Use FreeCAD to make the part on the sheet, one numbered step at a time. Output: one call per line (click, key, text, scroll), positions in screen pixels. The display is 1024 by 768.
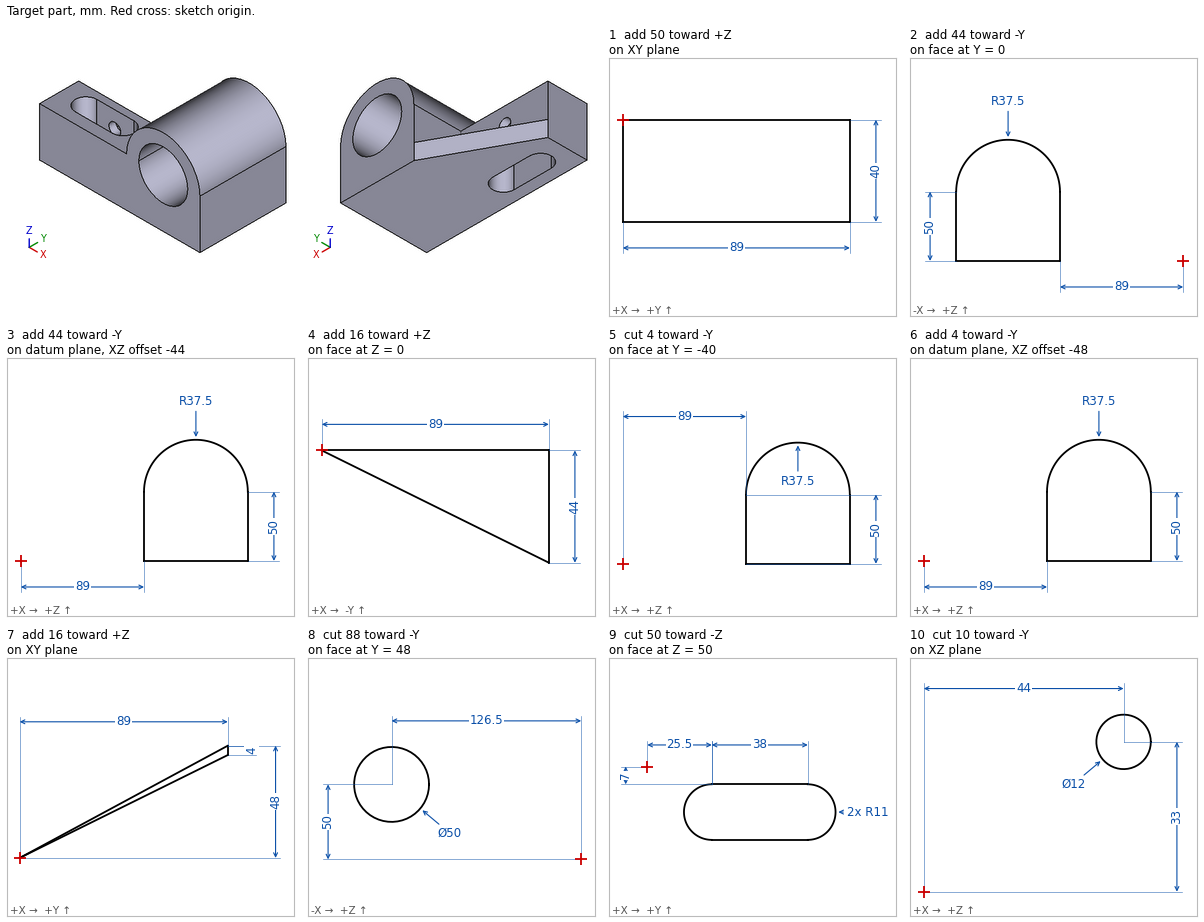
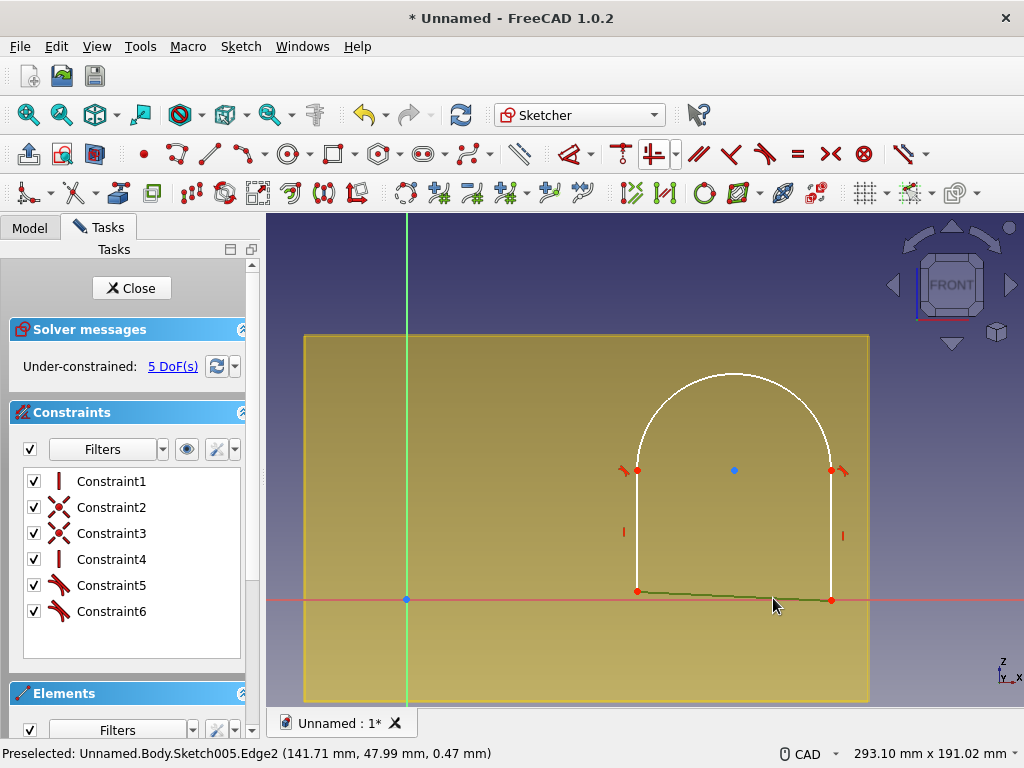
click(676, 154)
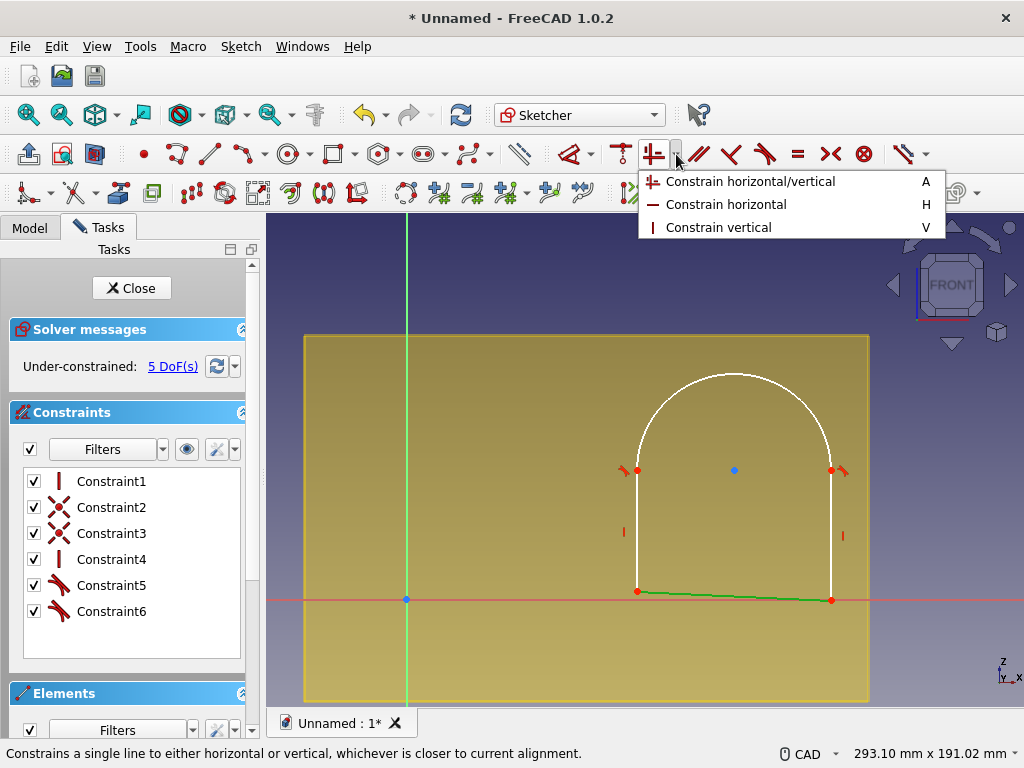
click(792, 204)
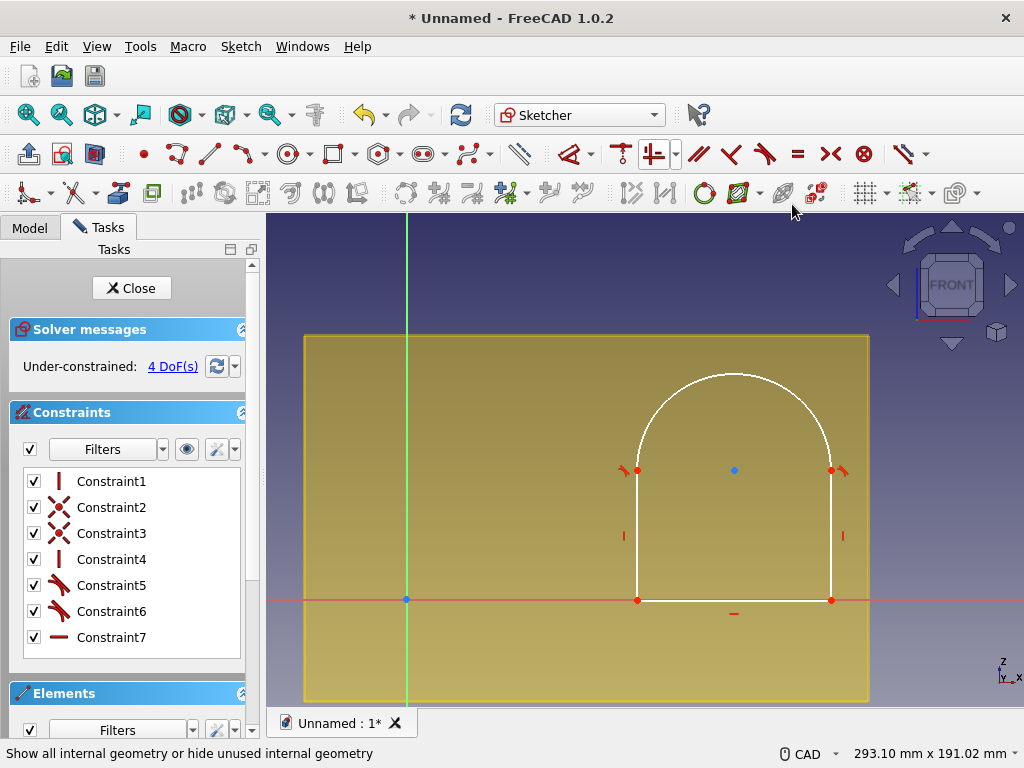
key(d)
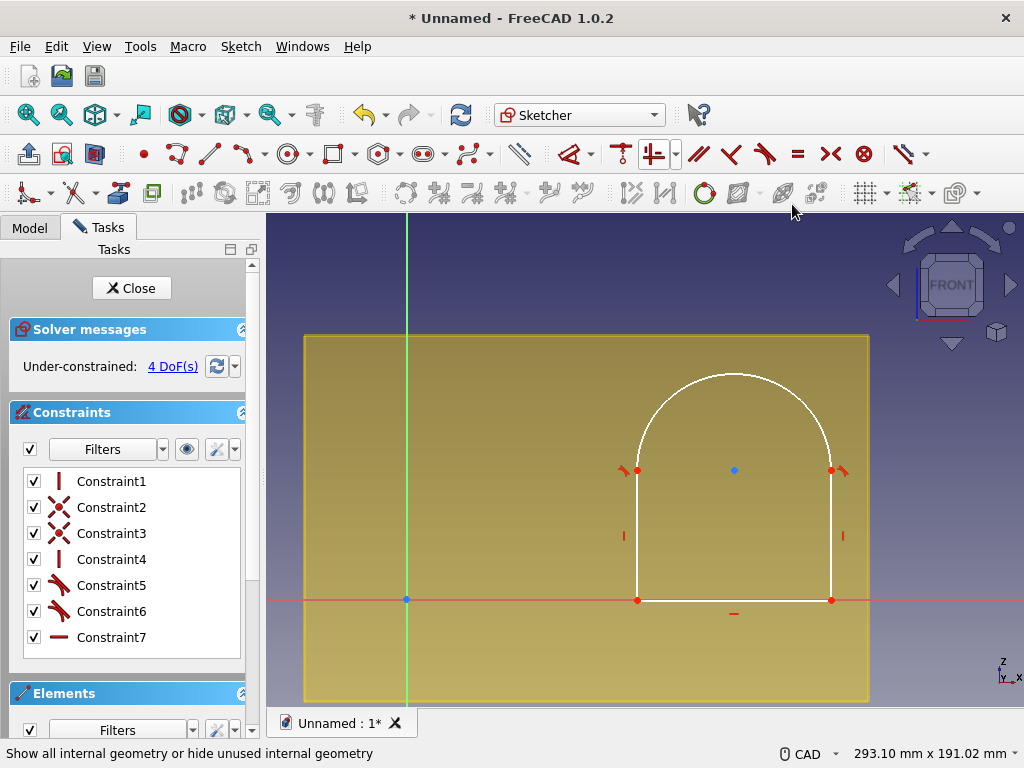
click(791, 393)
click(810, 367)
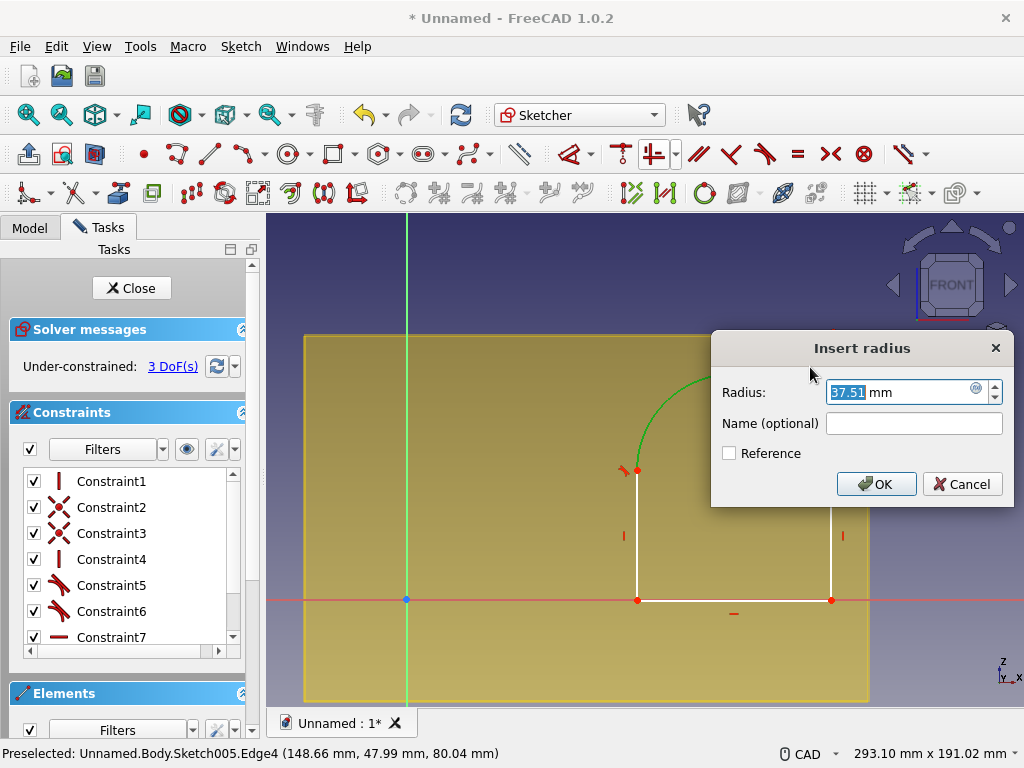
text(37.5)
key(Return)
key(Escape)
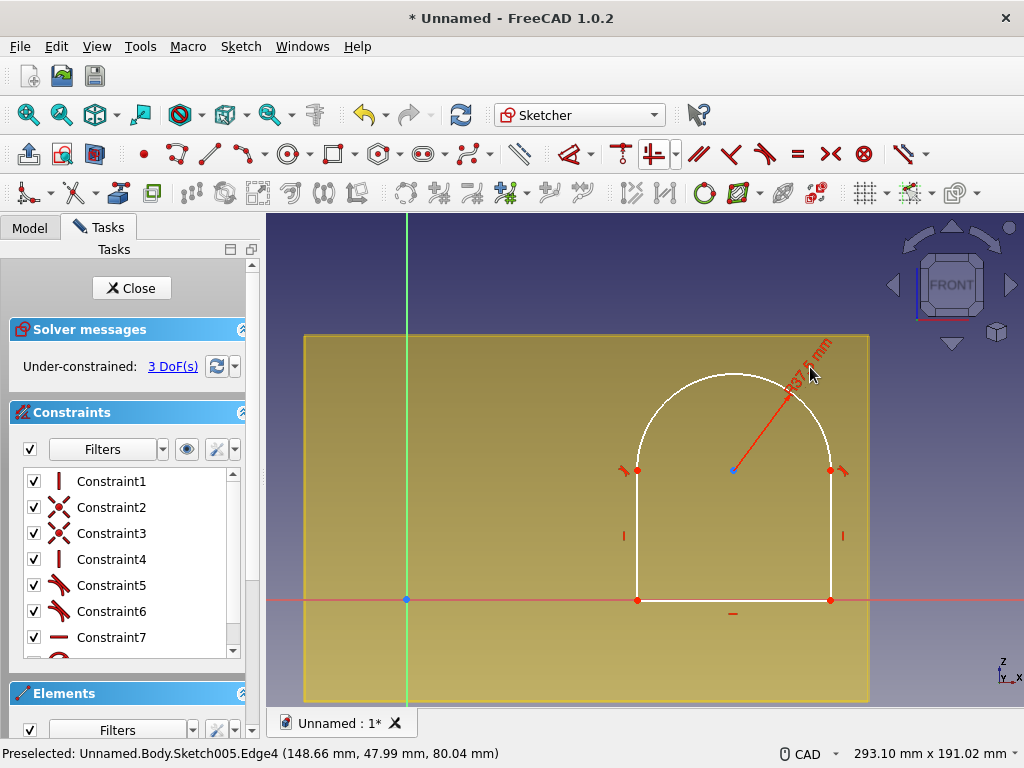
click(831, 601)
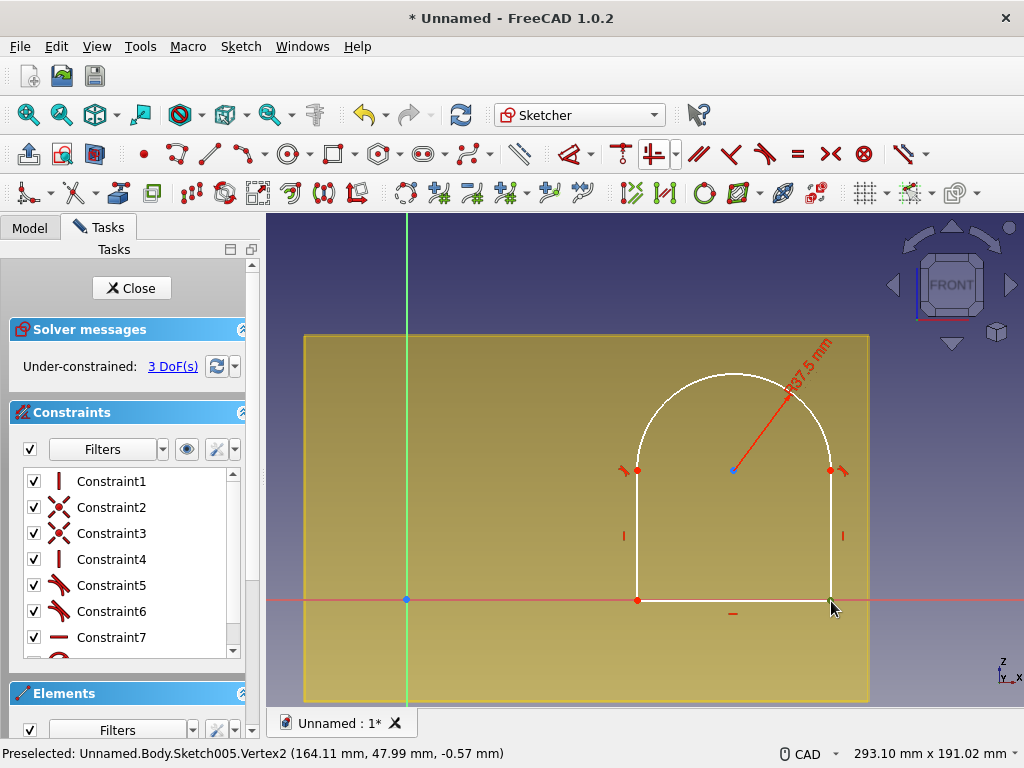
click(334, 600)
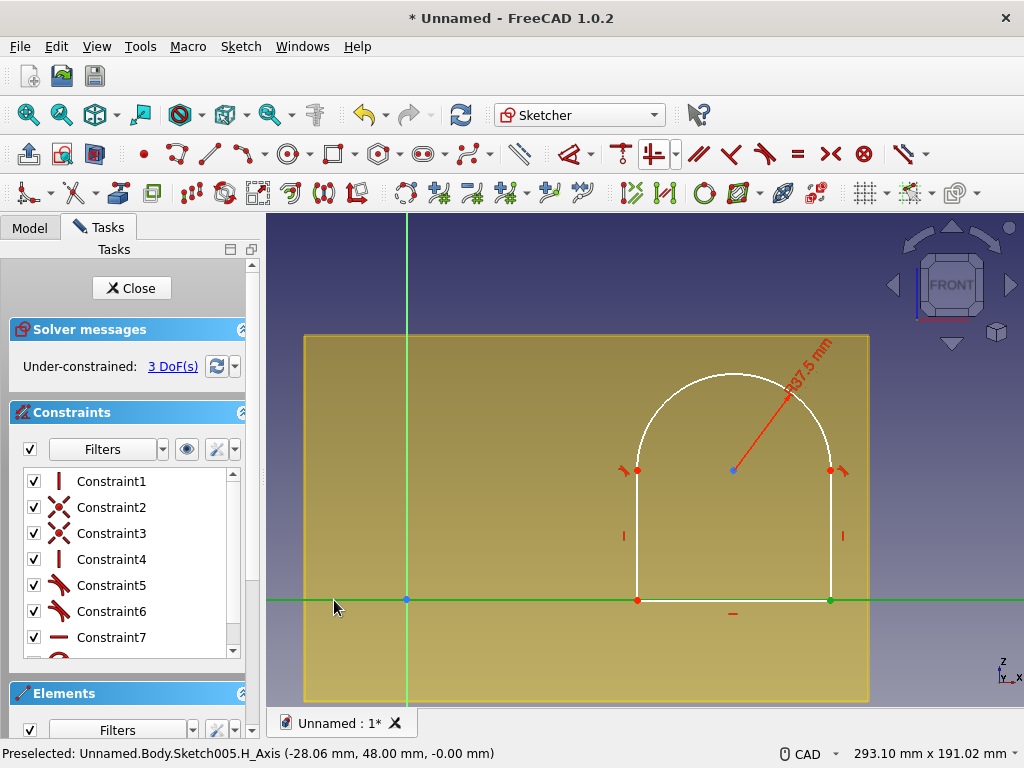
click(621, 154)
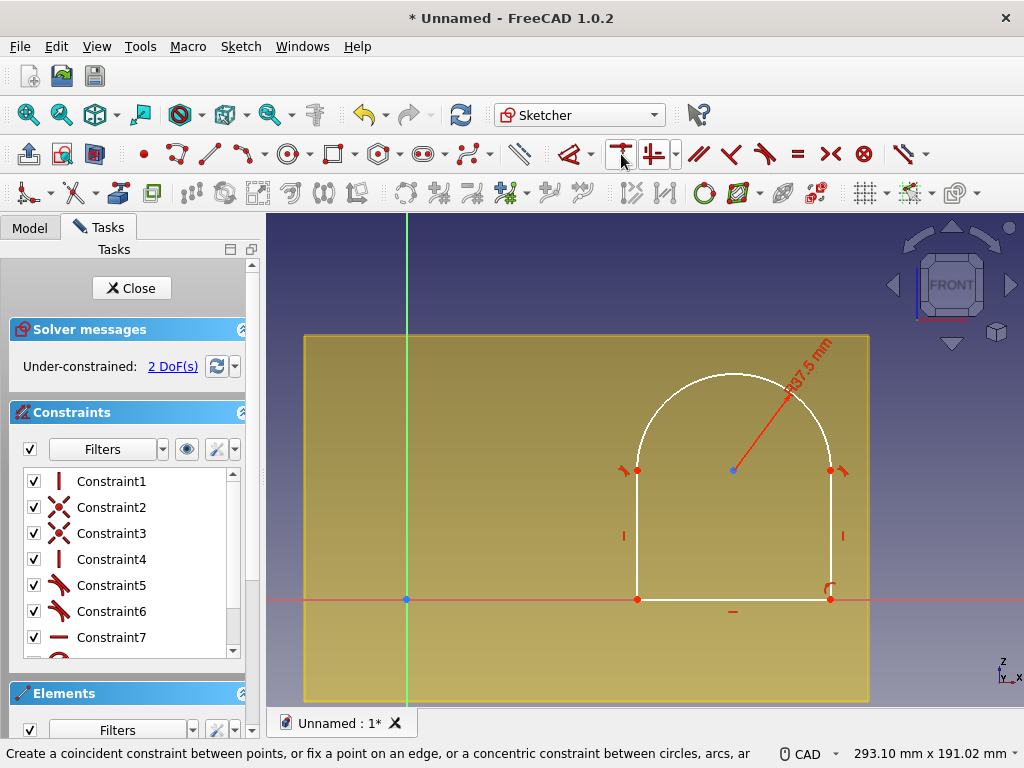
click(568, 154)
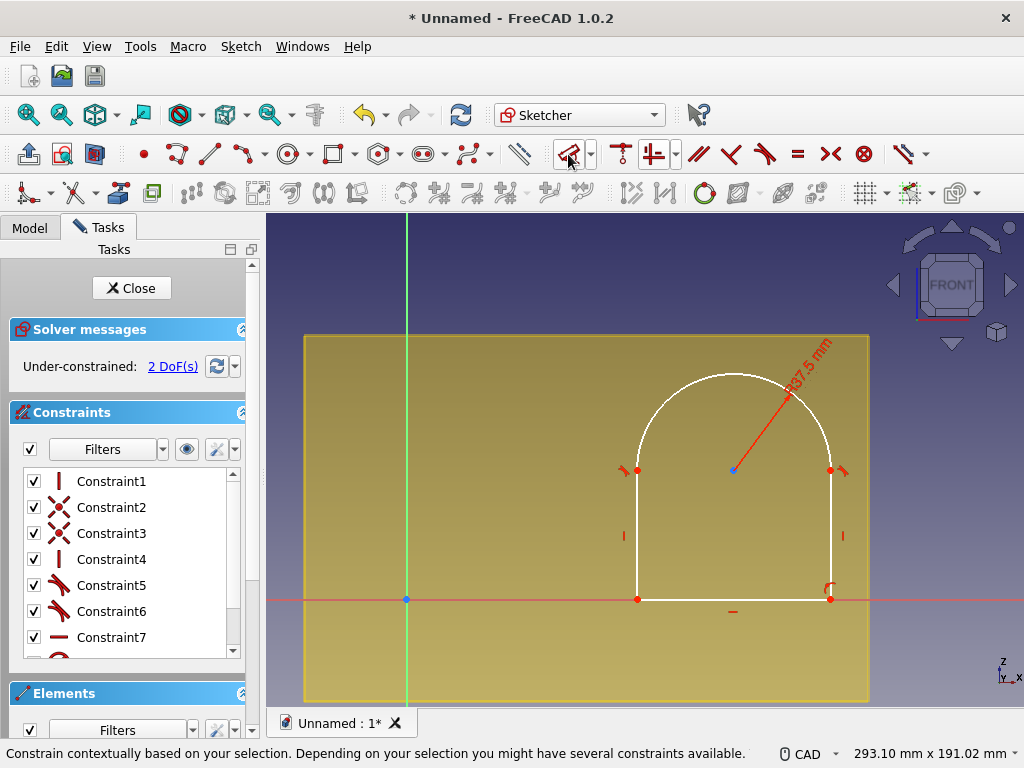
click(831, 510)
click(797, 535)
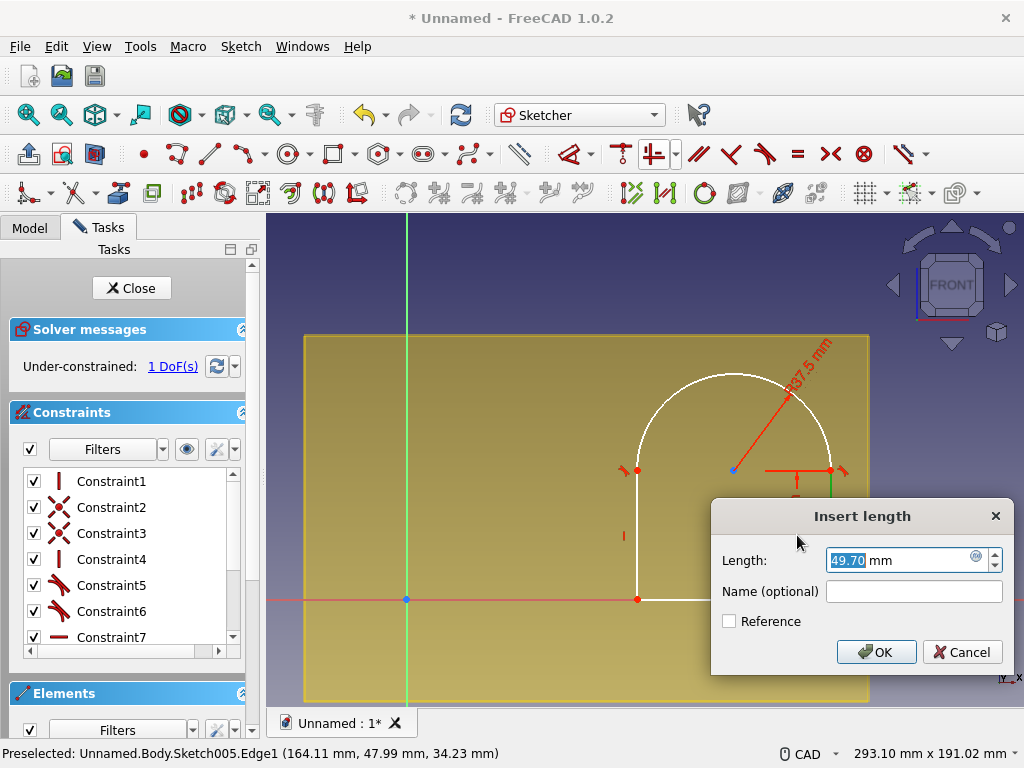
text(50)
key(Return)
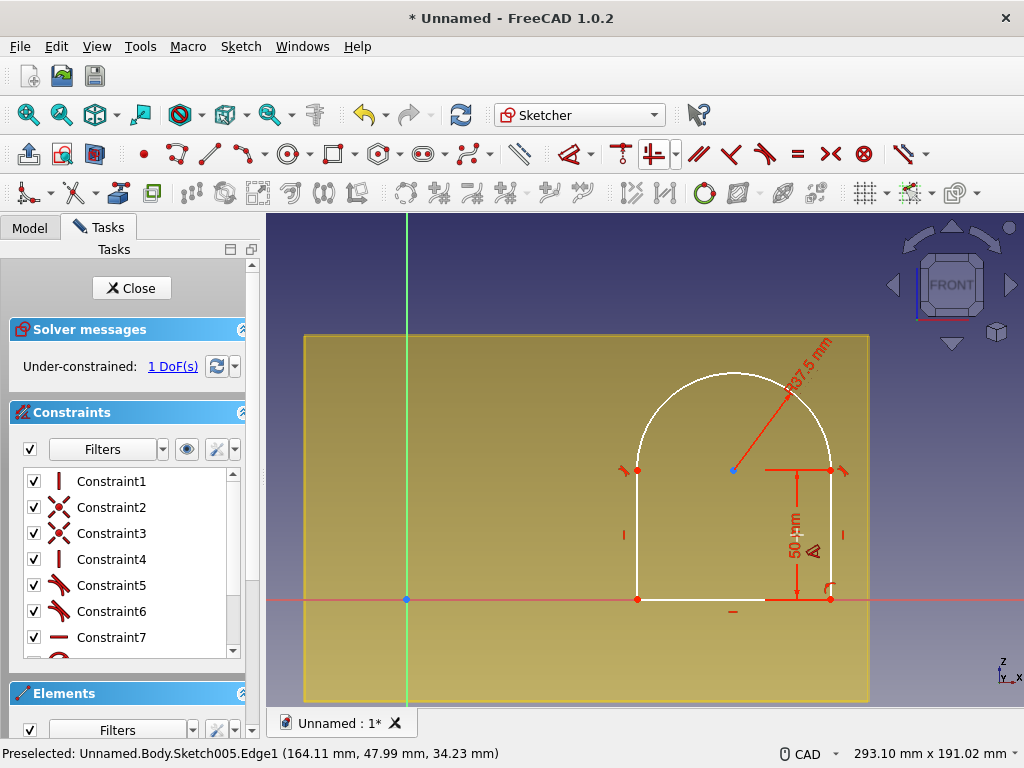
click(637, 600)
click(522, 634)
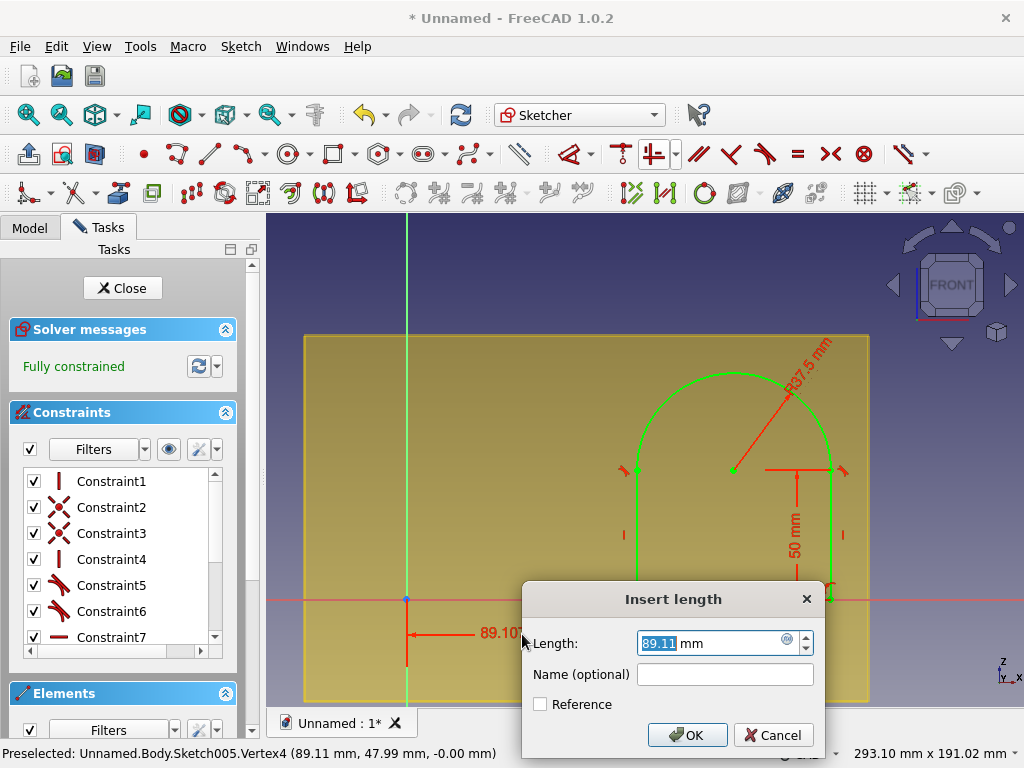
text(89)
key(Return)
key(Escape)